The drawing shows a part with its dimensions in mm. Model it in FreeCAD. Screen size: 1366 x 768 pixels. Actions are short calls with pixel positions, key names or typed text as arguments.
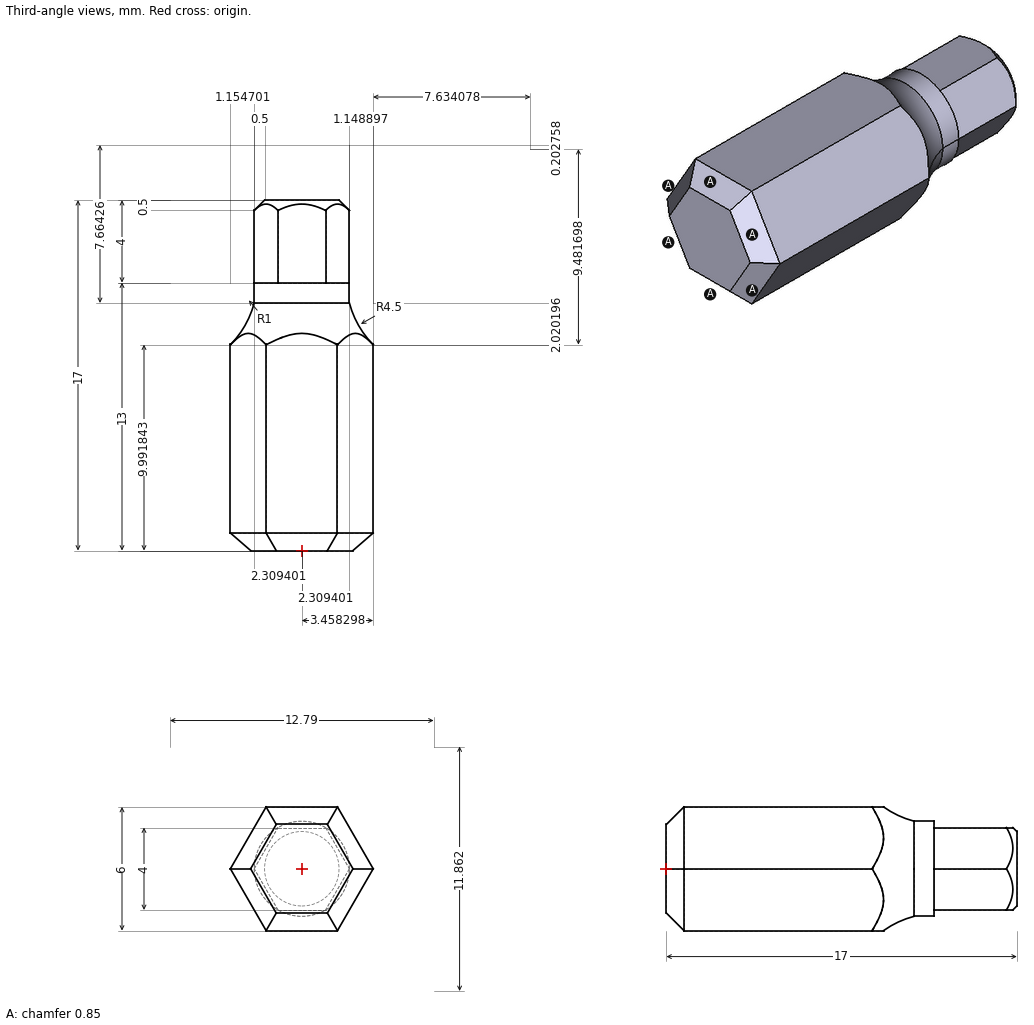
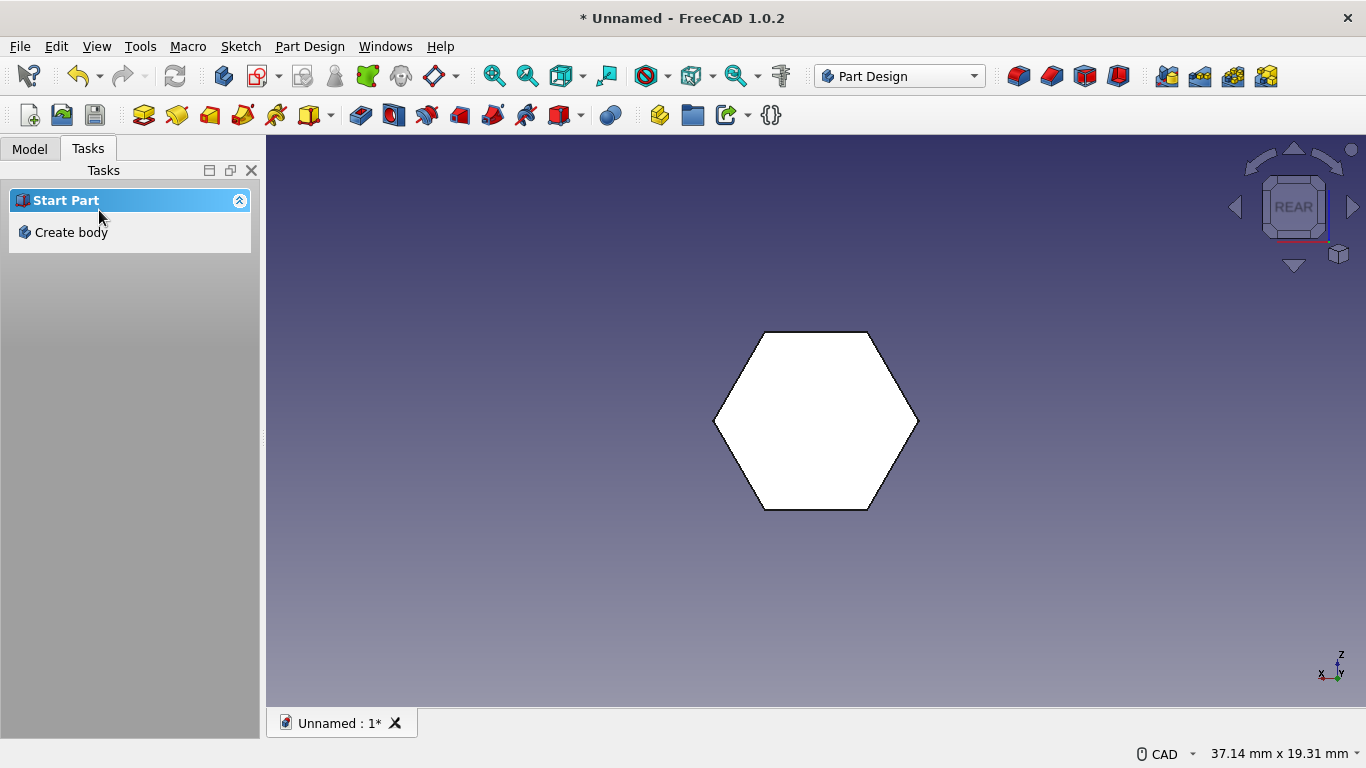
click(495, 76)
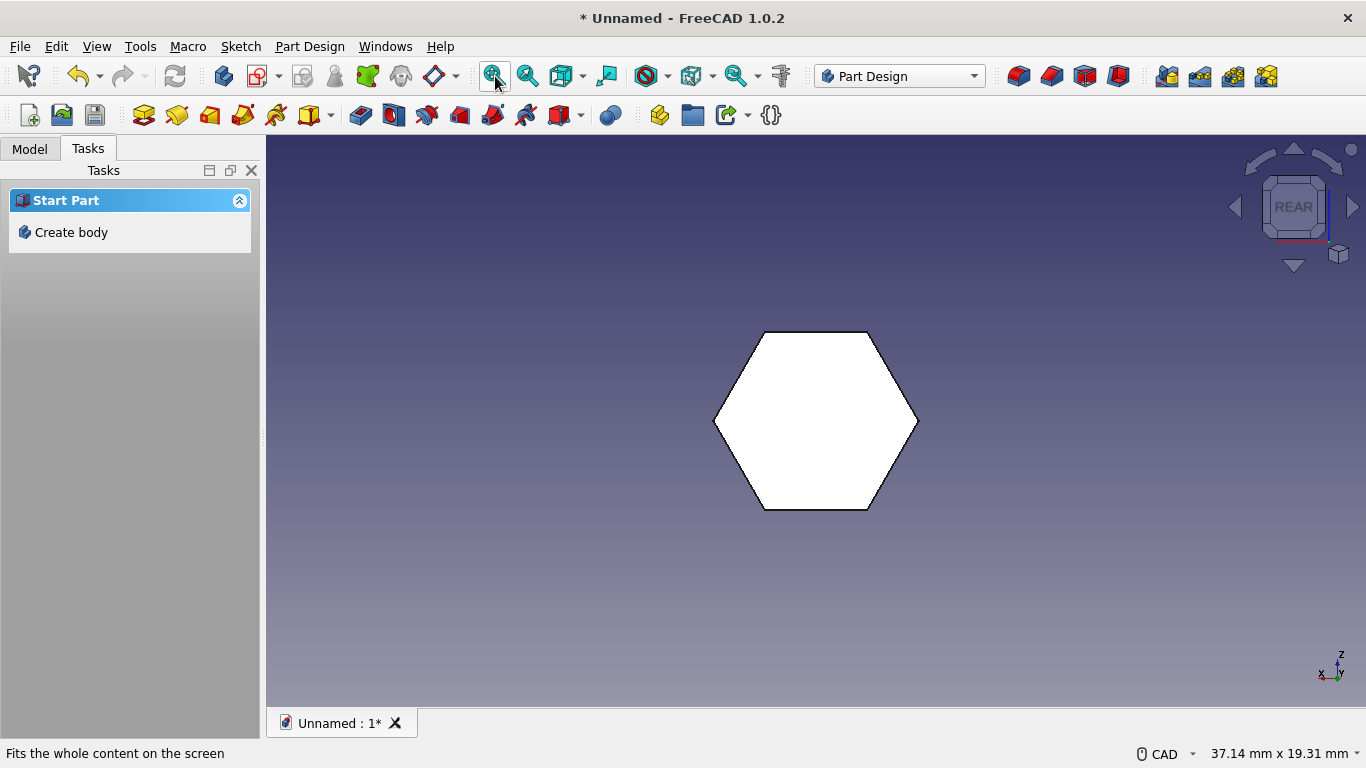
click(816, 420)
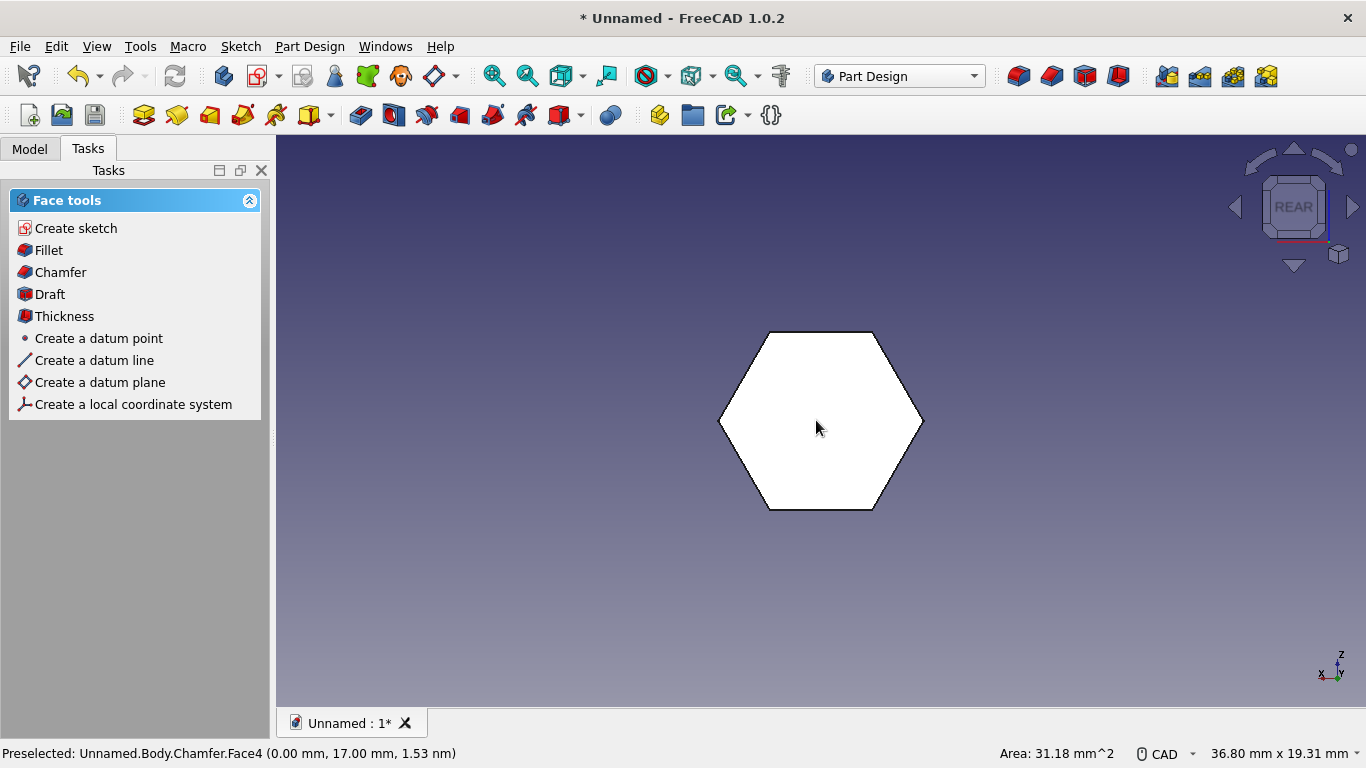
click(256, 76)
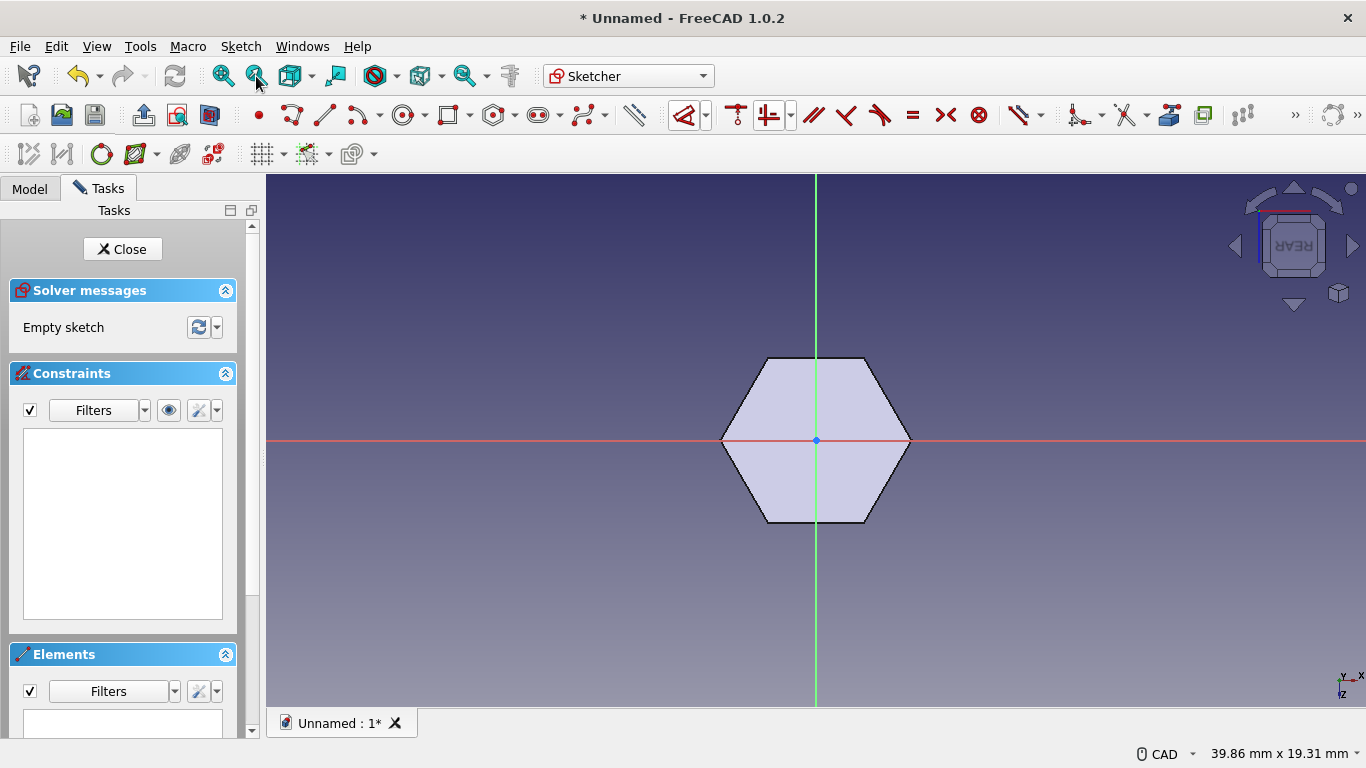
click(470, 116)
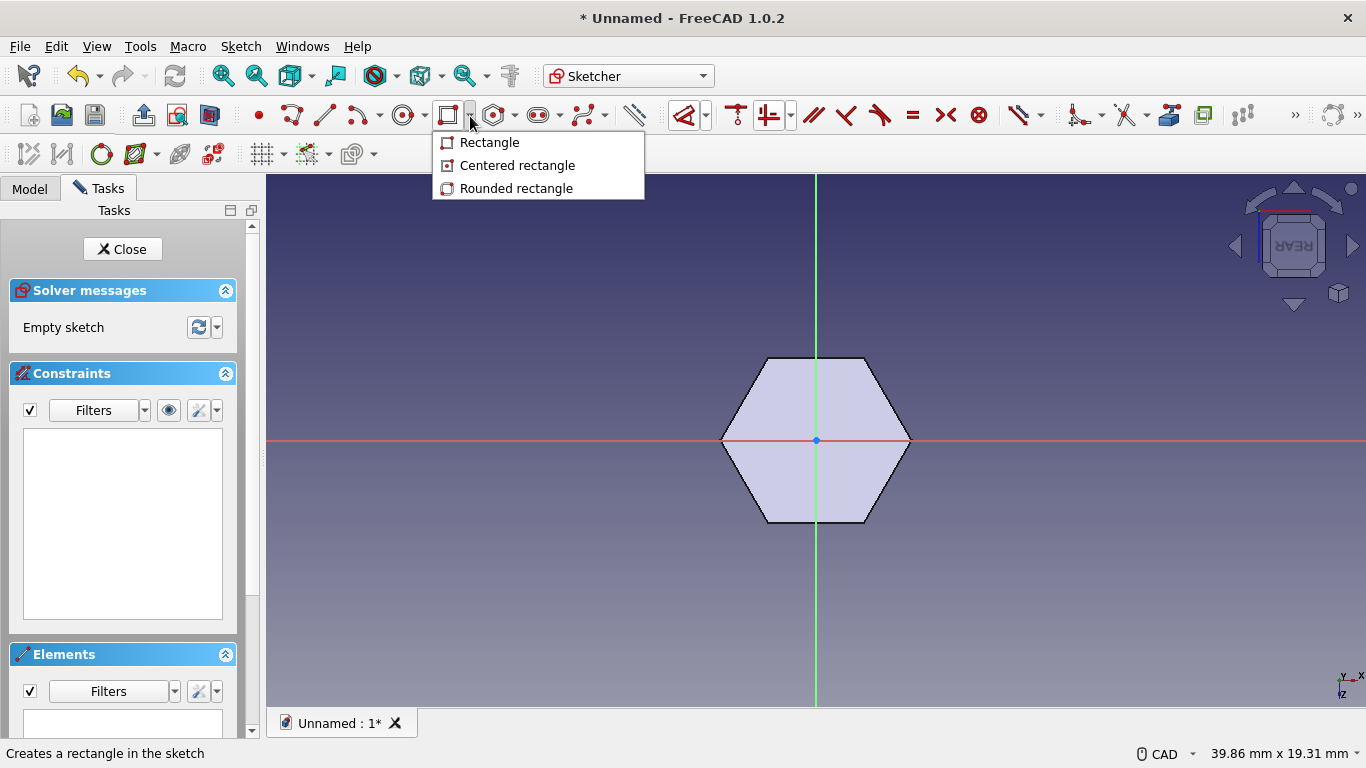
click(538, 166)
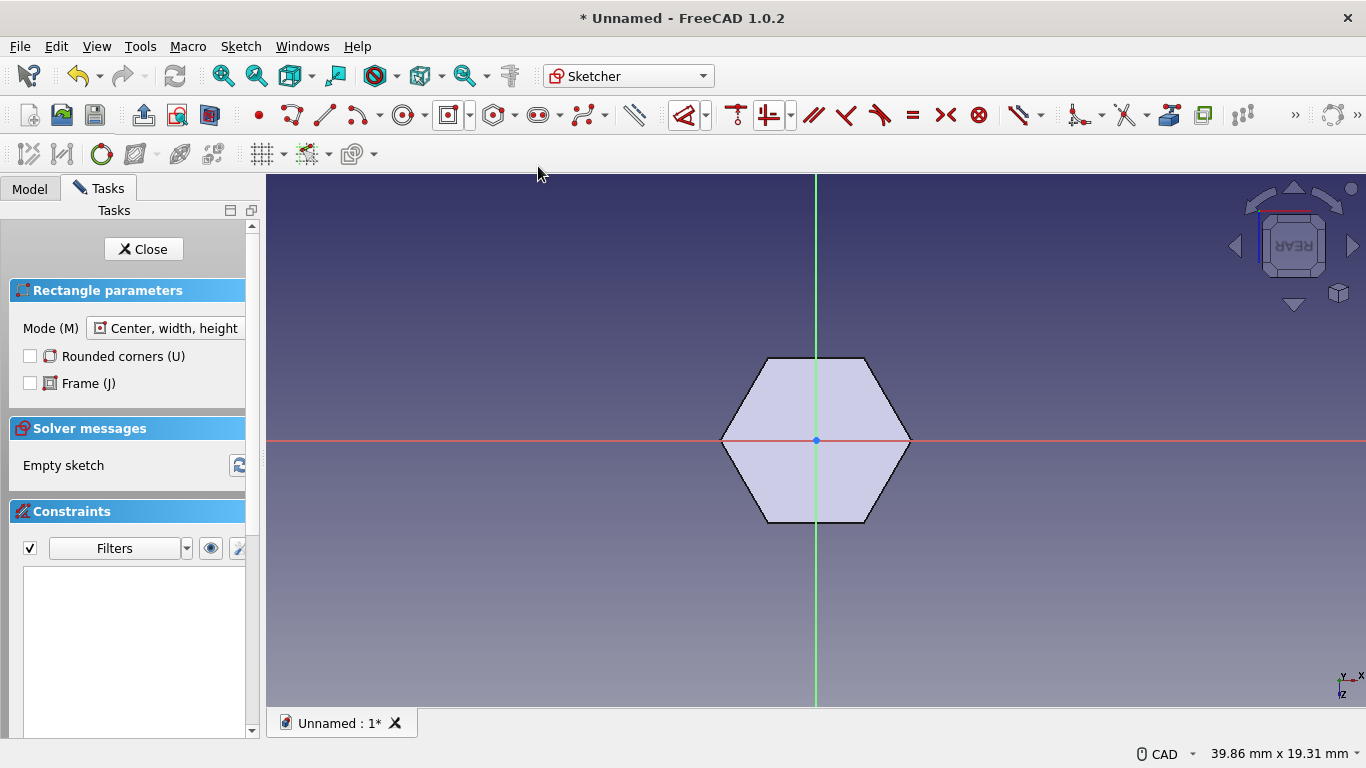
click(816, 440)
click(992, 277)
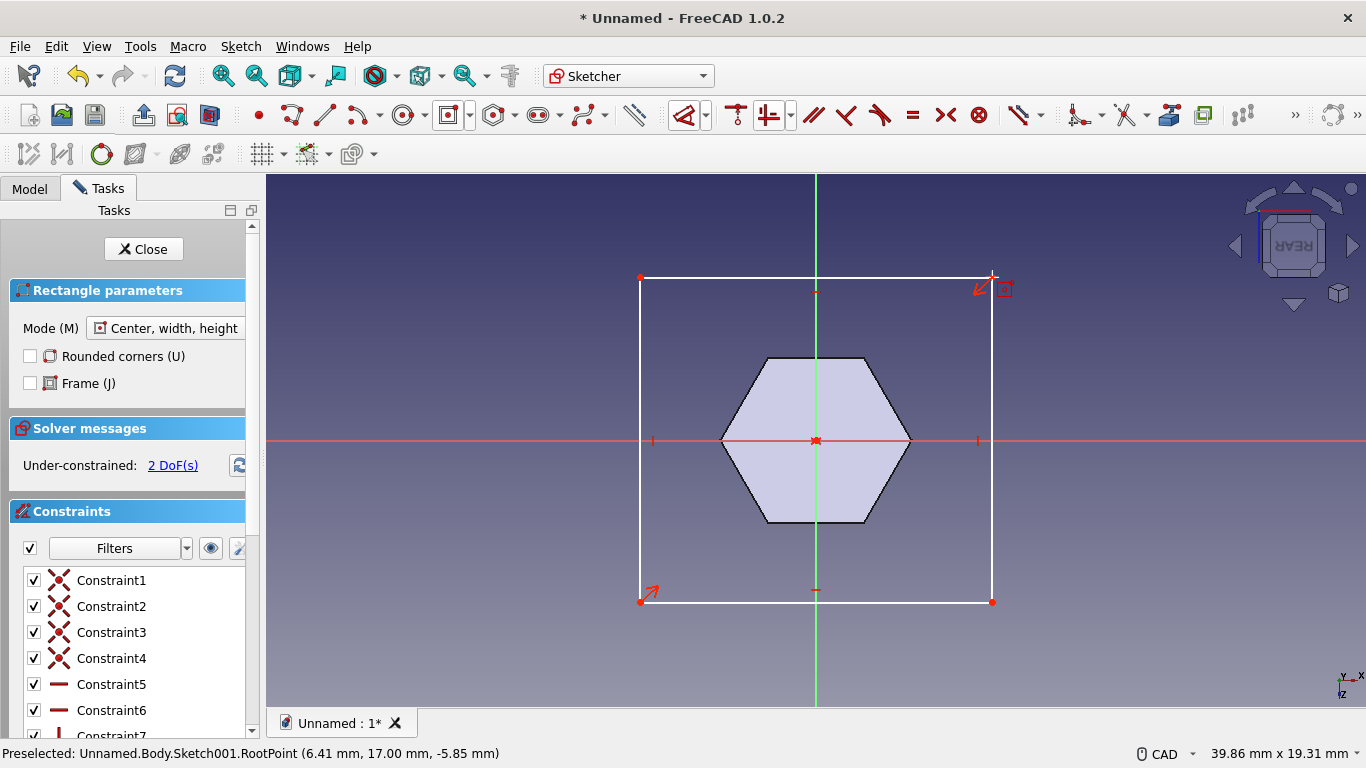
click(492, 116)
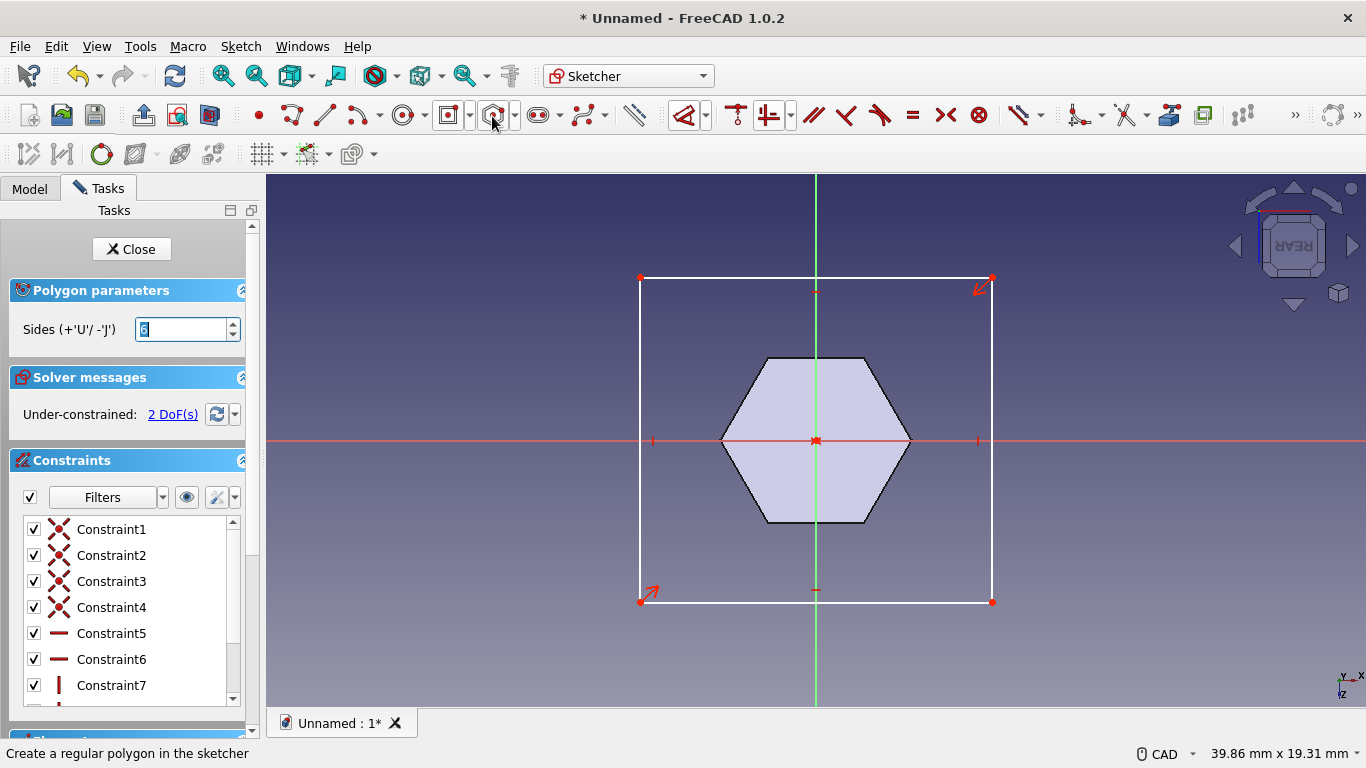
click(816, 440)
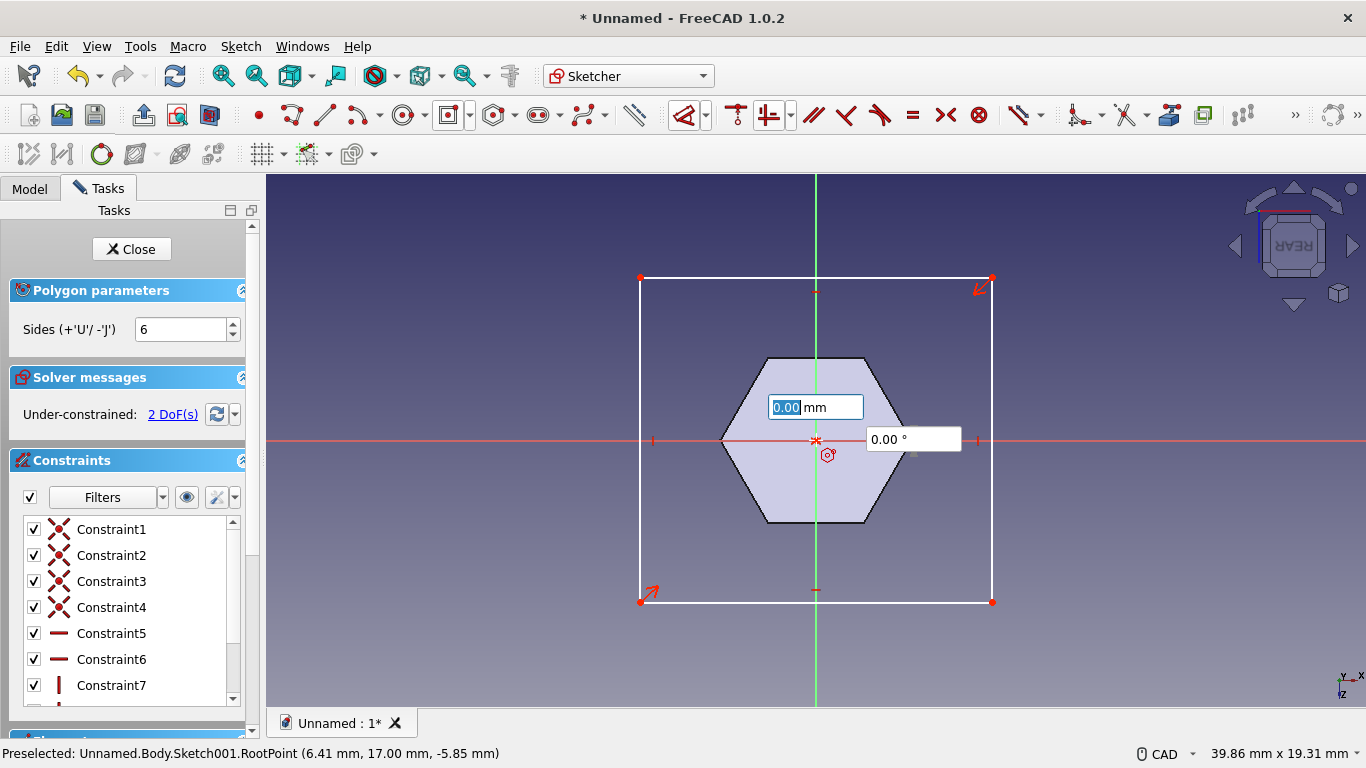
click(880, 440)
key(Escape)